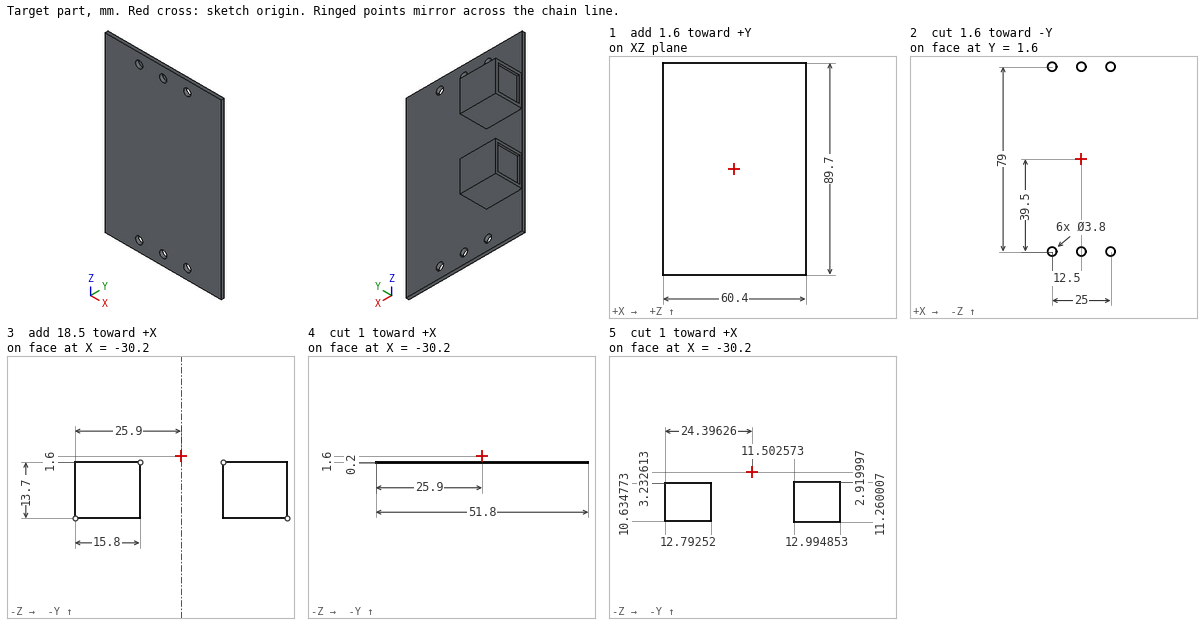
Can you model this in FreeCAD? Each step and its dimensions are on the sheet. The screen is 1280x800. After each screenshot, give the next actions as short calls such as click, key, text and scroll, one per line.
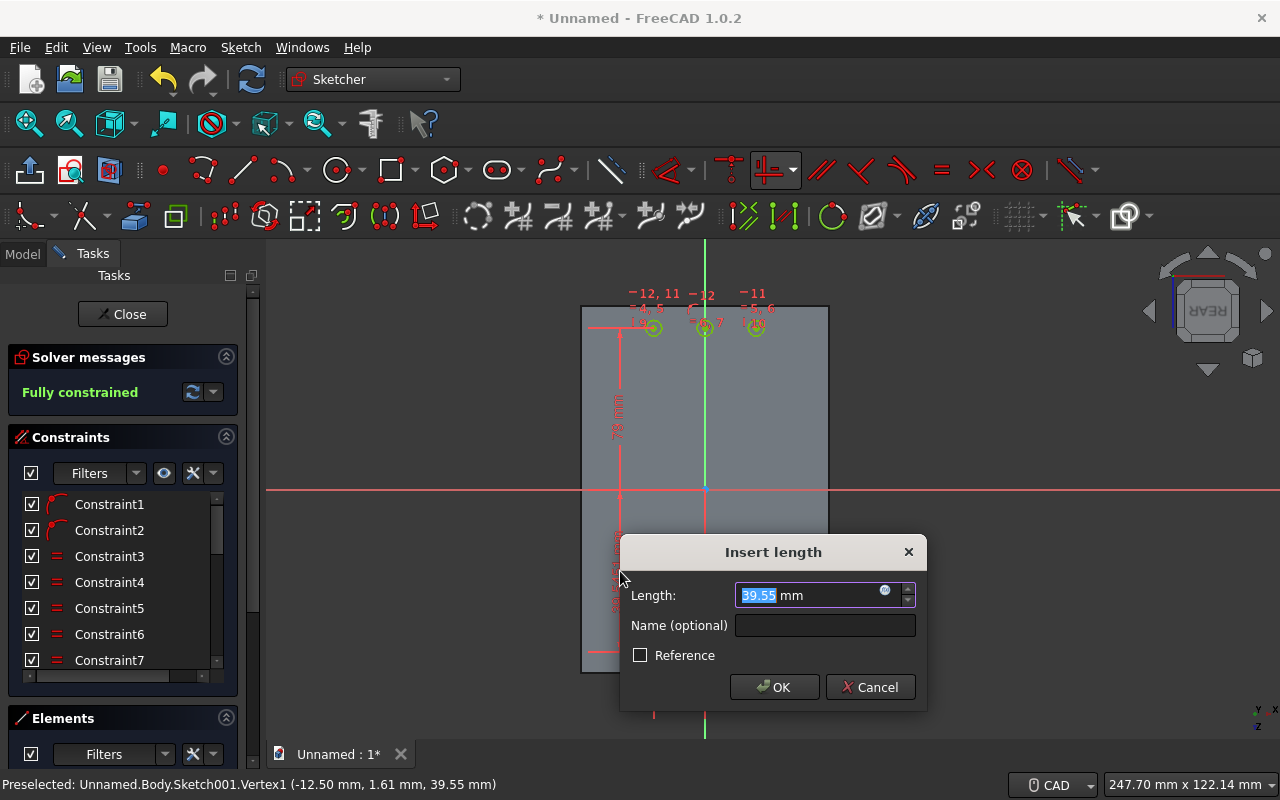
text(39.5)
key(Return)
key(Escape)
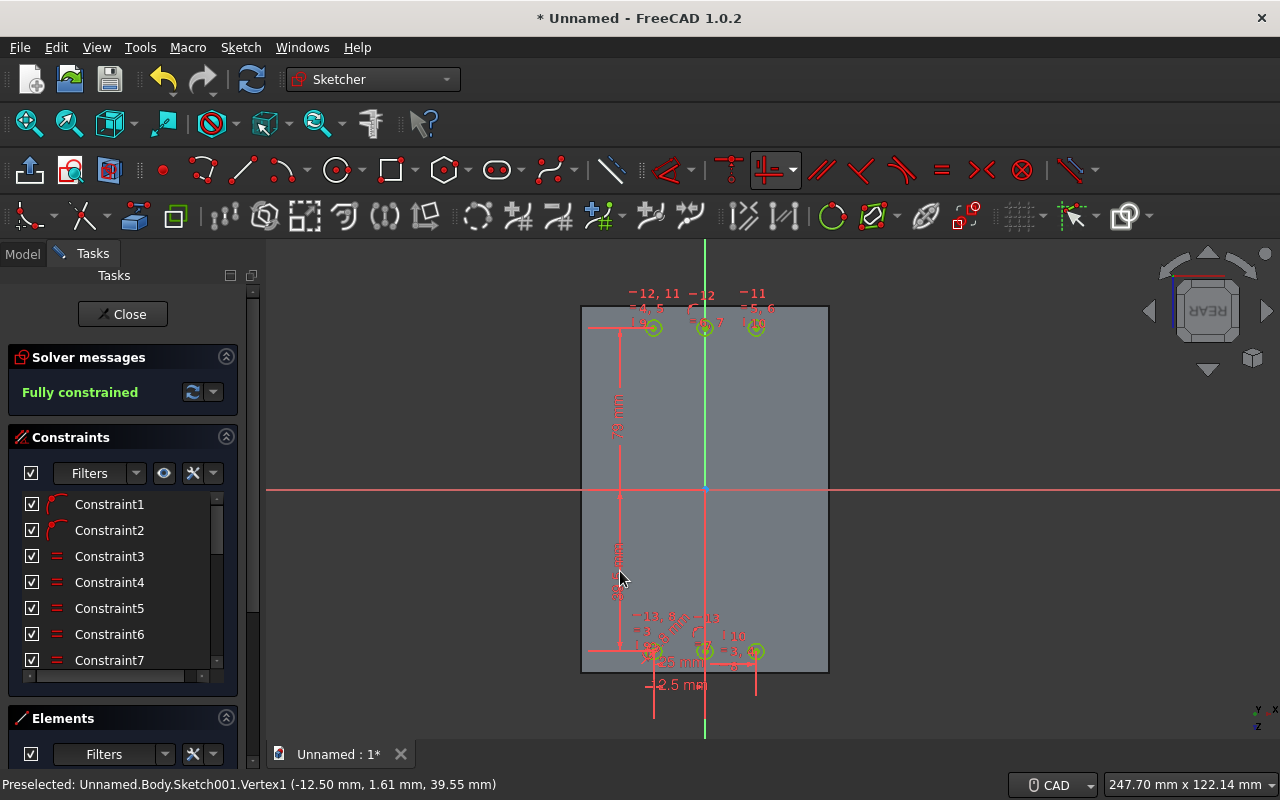
click(123, 314)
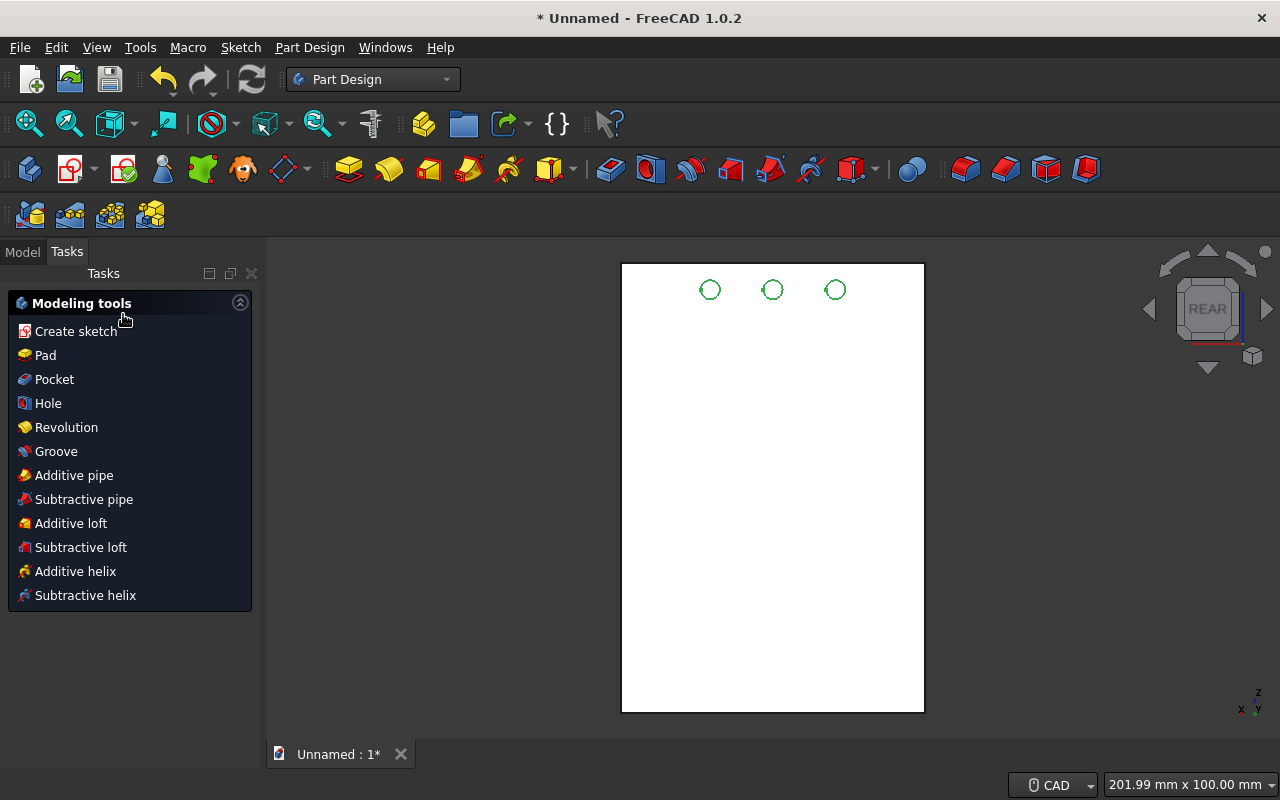
click(612, 170)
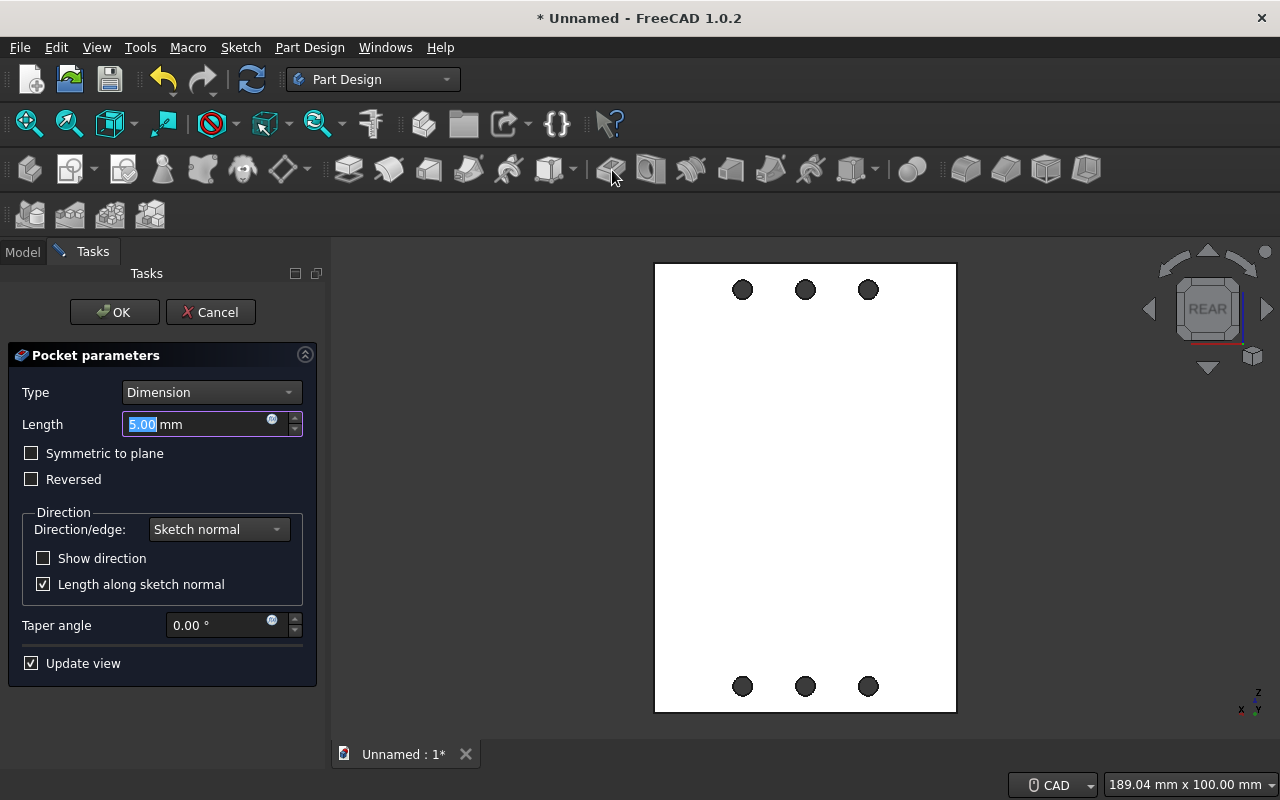
text(1.6)
key(Tab)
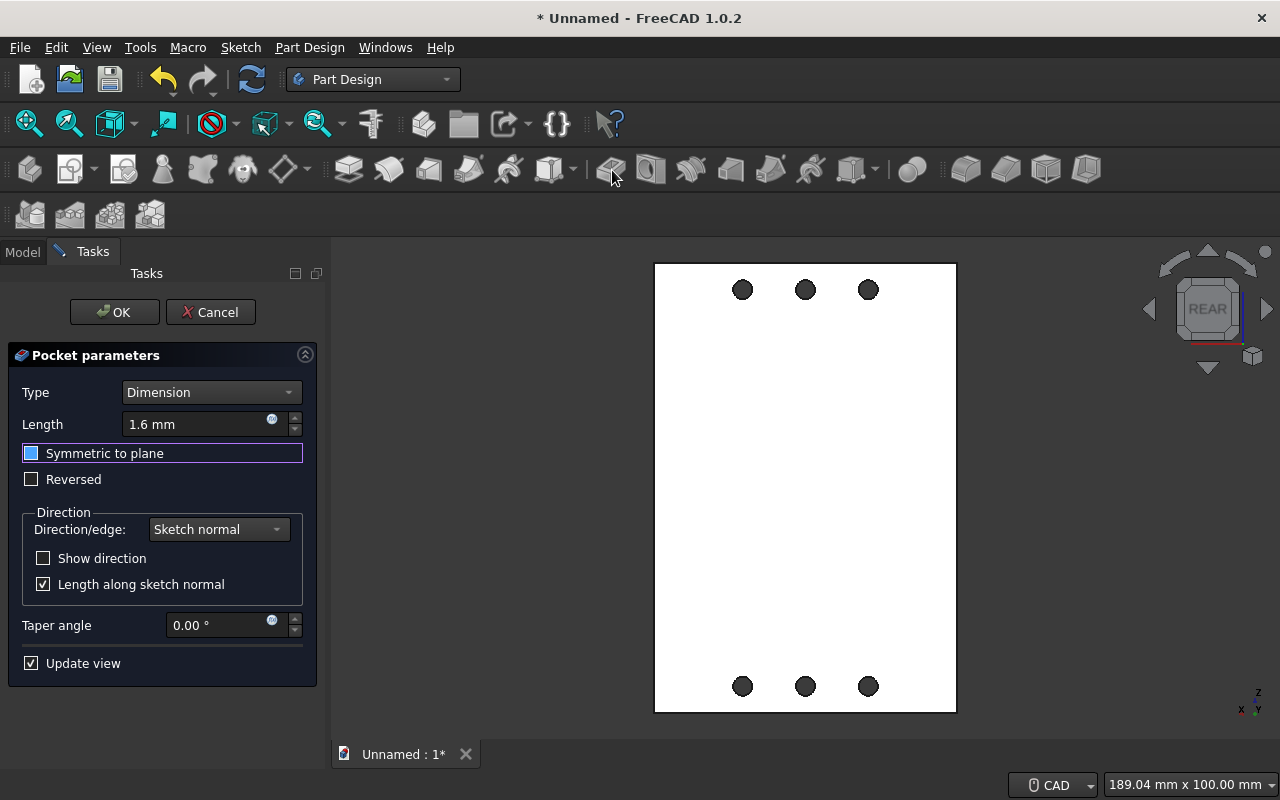
click(115, 312)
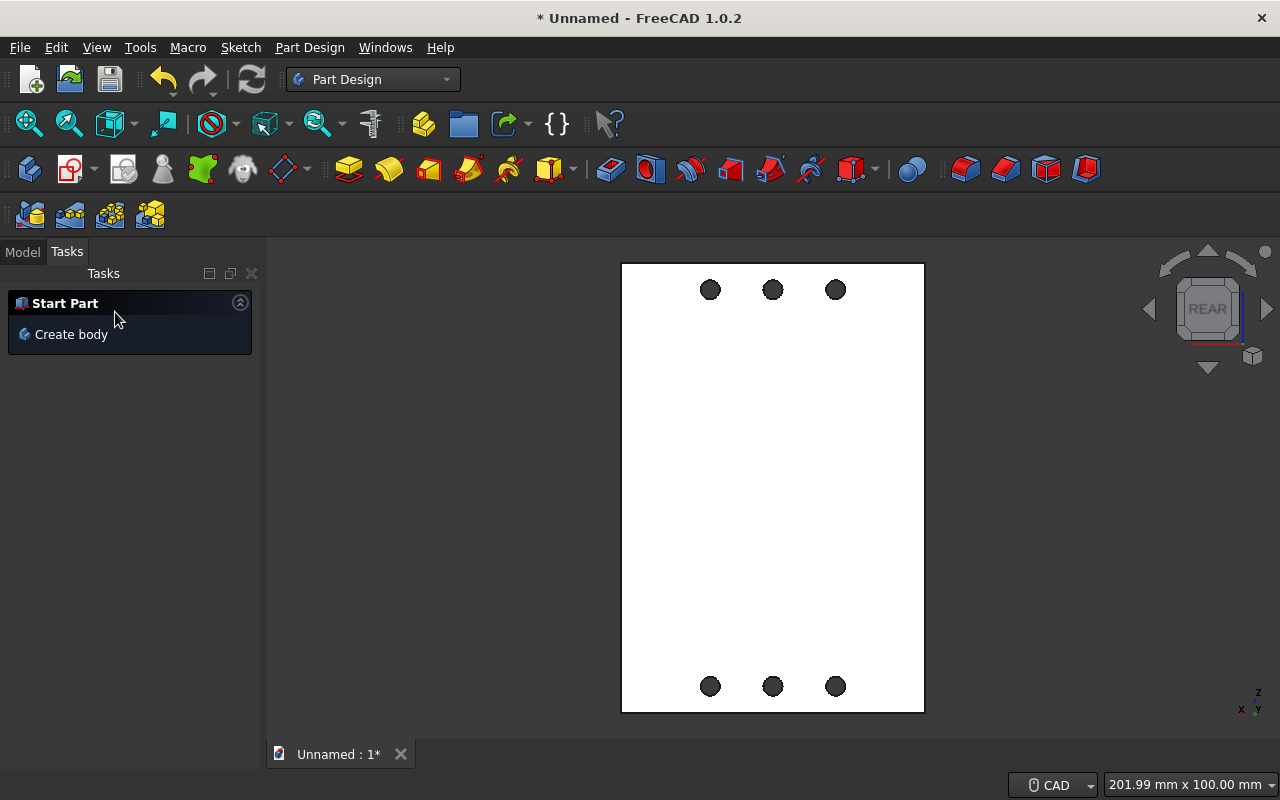
key(6)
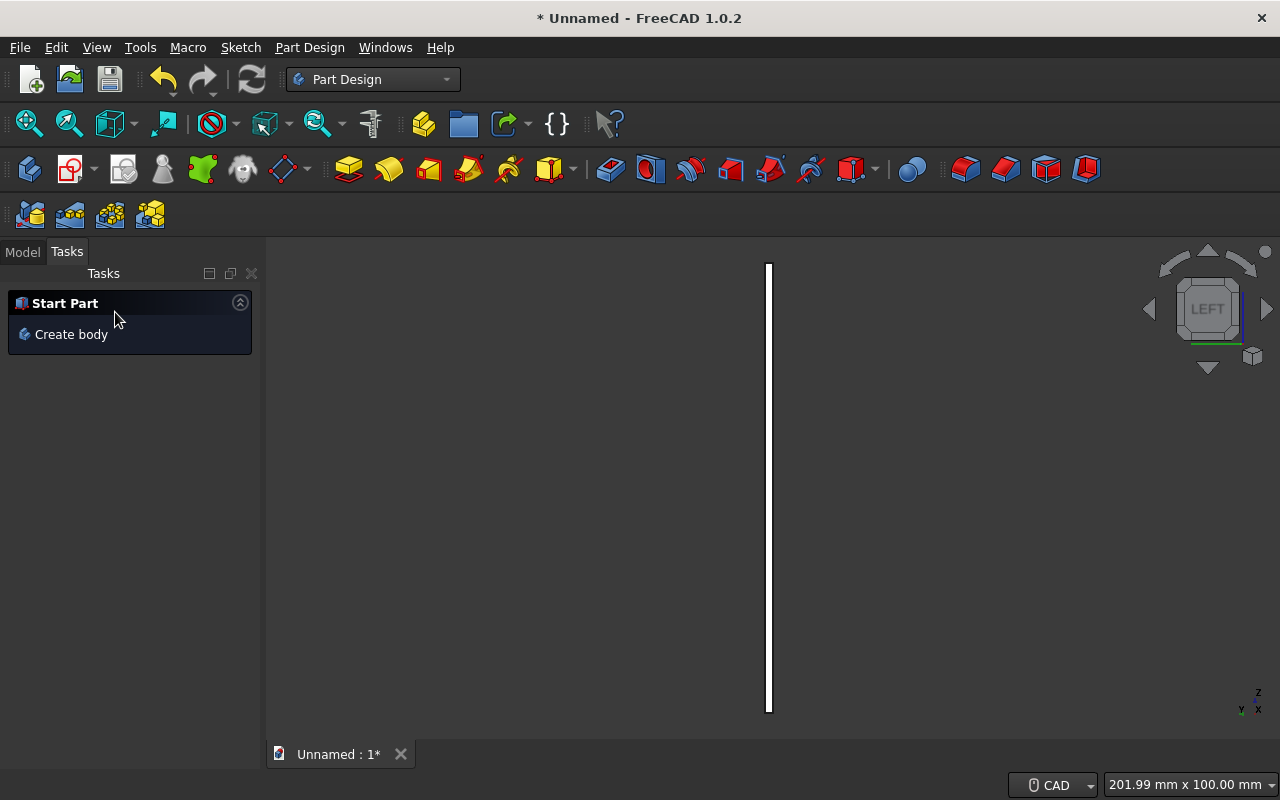
scroll(769, 358, up, 6)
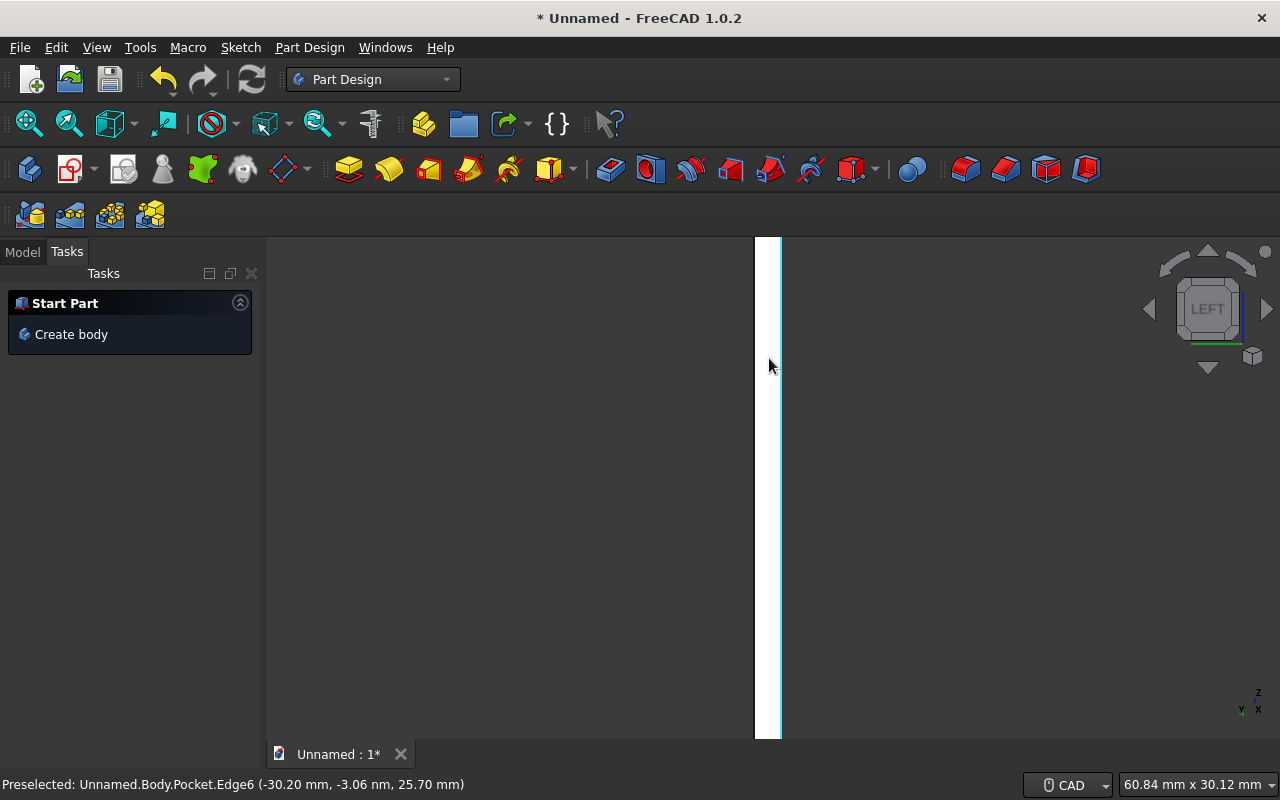
click(768, 361)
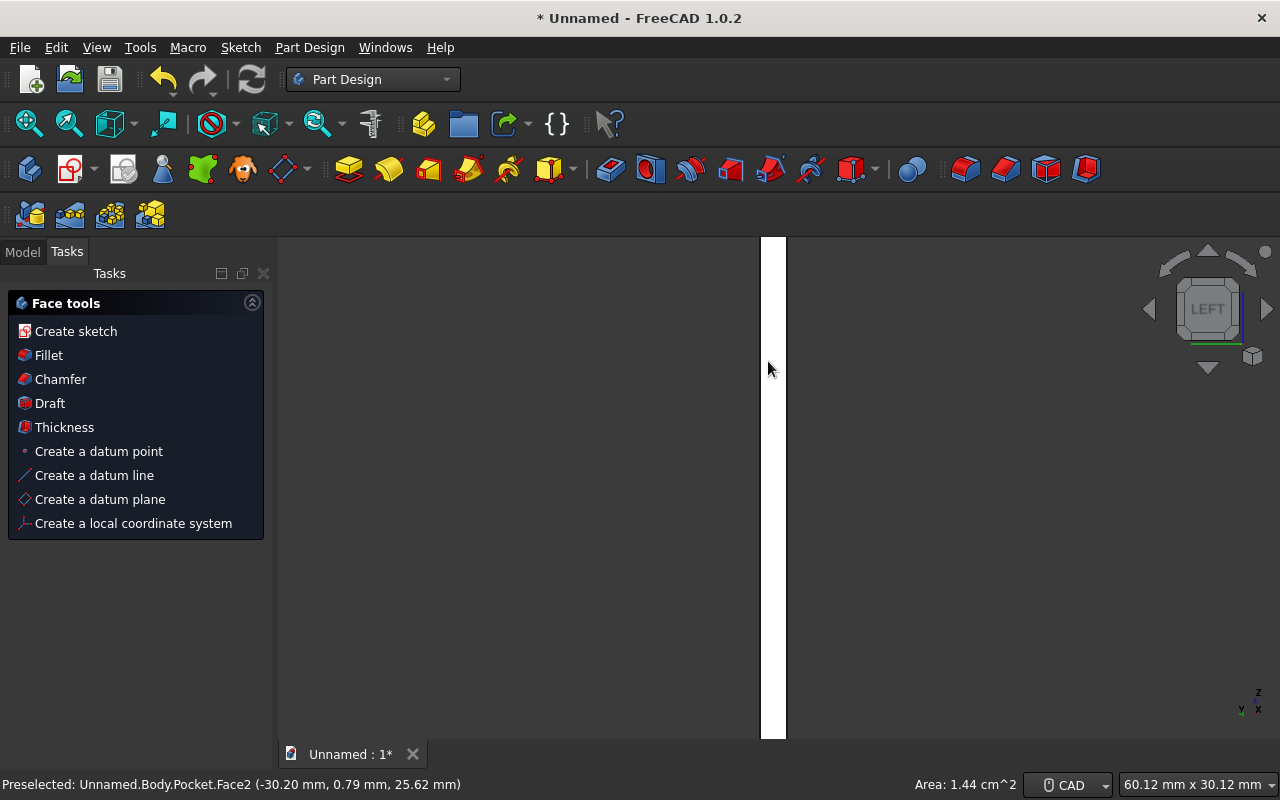
click(70, 170)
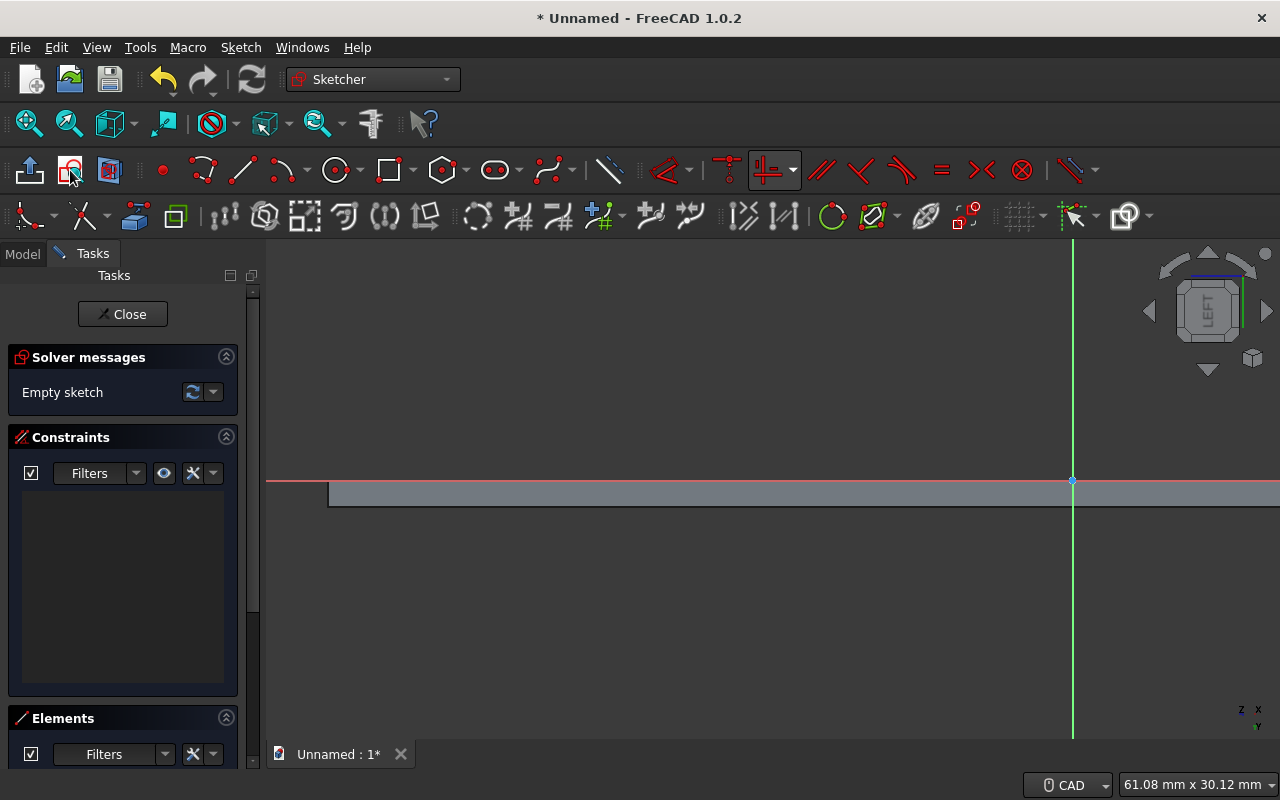
scroll(294, 344, down, 3)